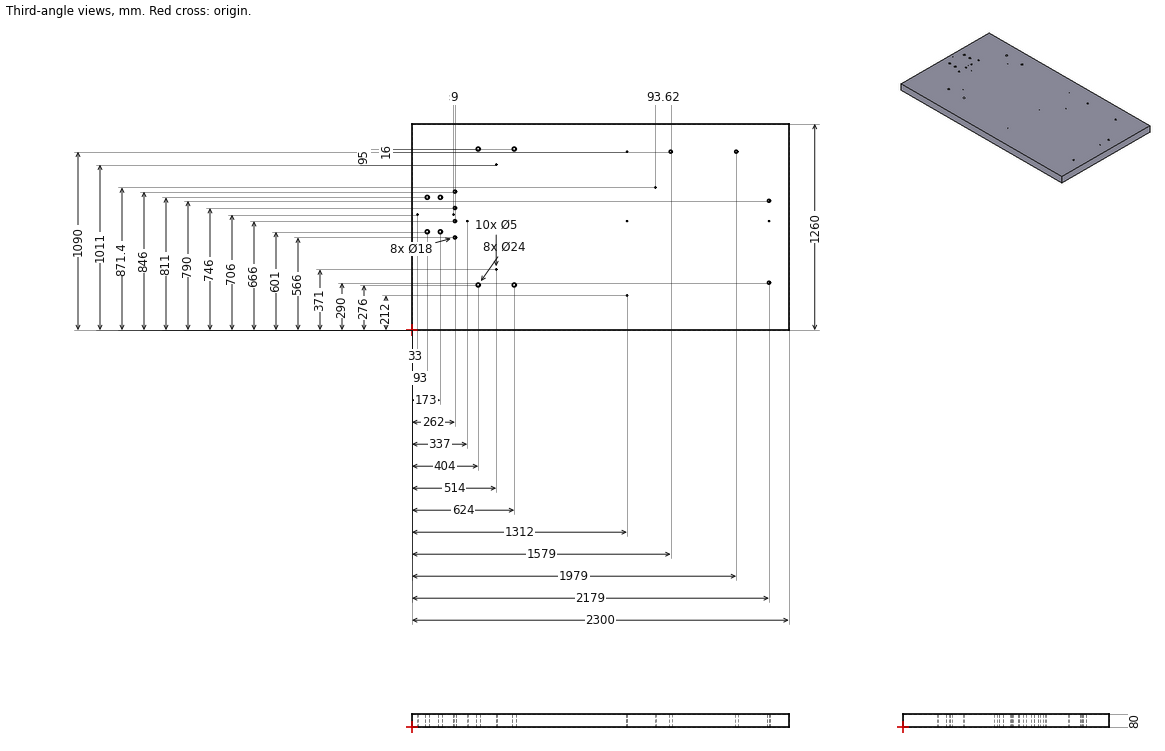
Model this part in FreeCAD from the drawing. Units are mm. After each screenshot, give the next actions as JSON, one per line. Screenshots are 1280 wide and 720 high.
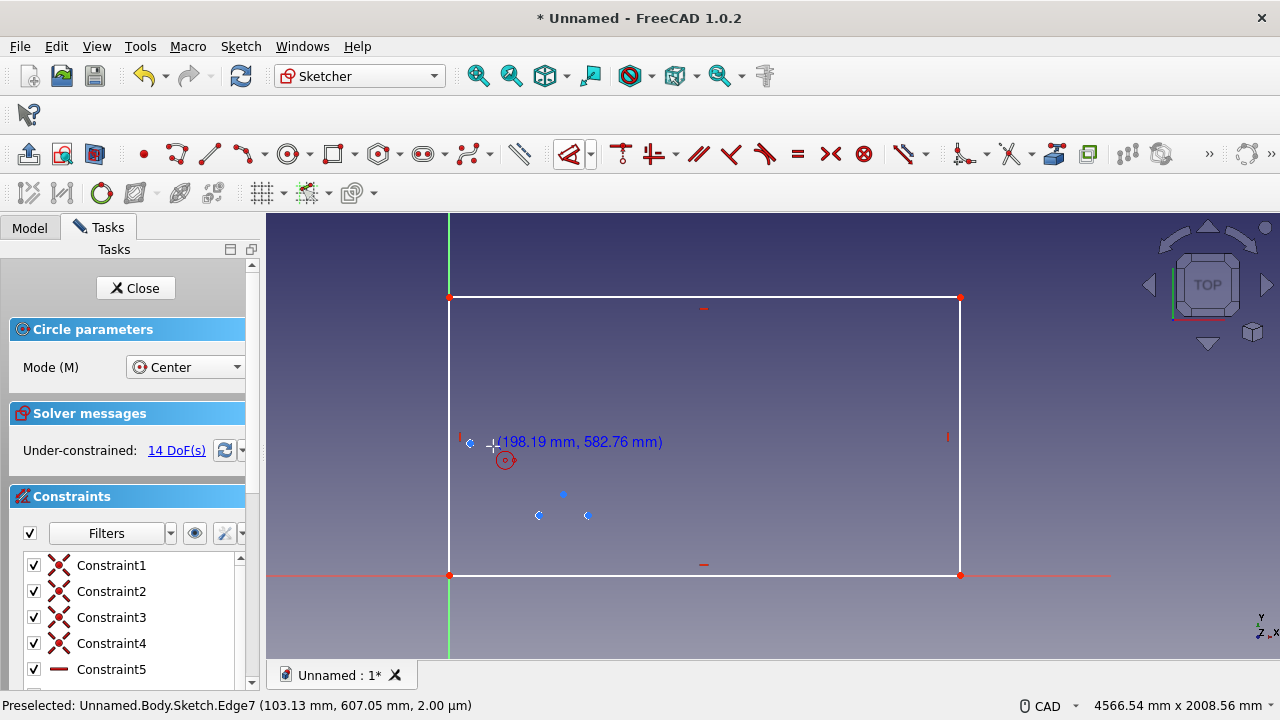
{"action": "left_click", "coordinate": [507, 450]}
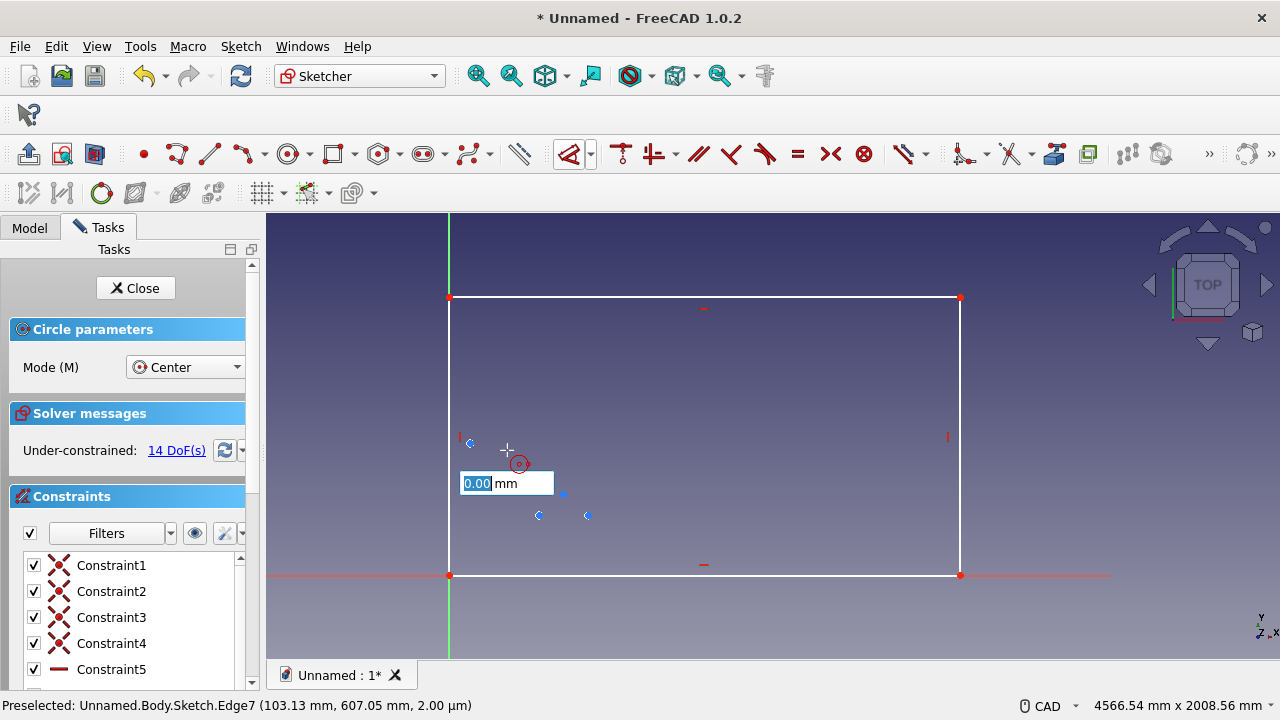
{"action": "scroll", "coordinate": [509, 449], "scroll_direction": "up", "scroll_amount": 11}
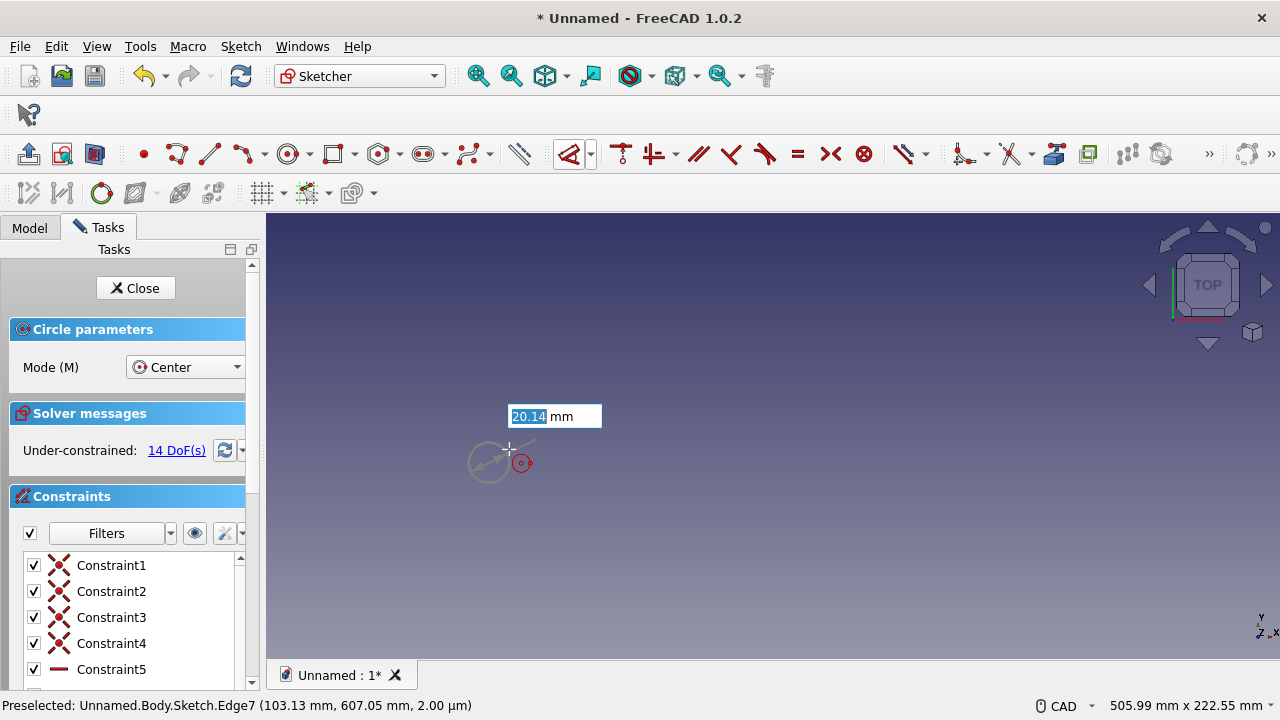
{"action": "left_click", "coordinate": [505, 444]}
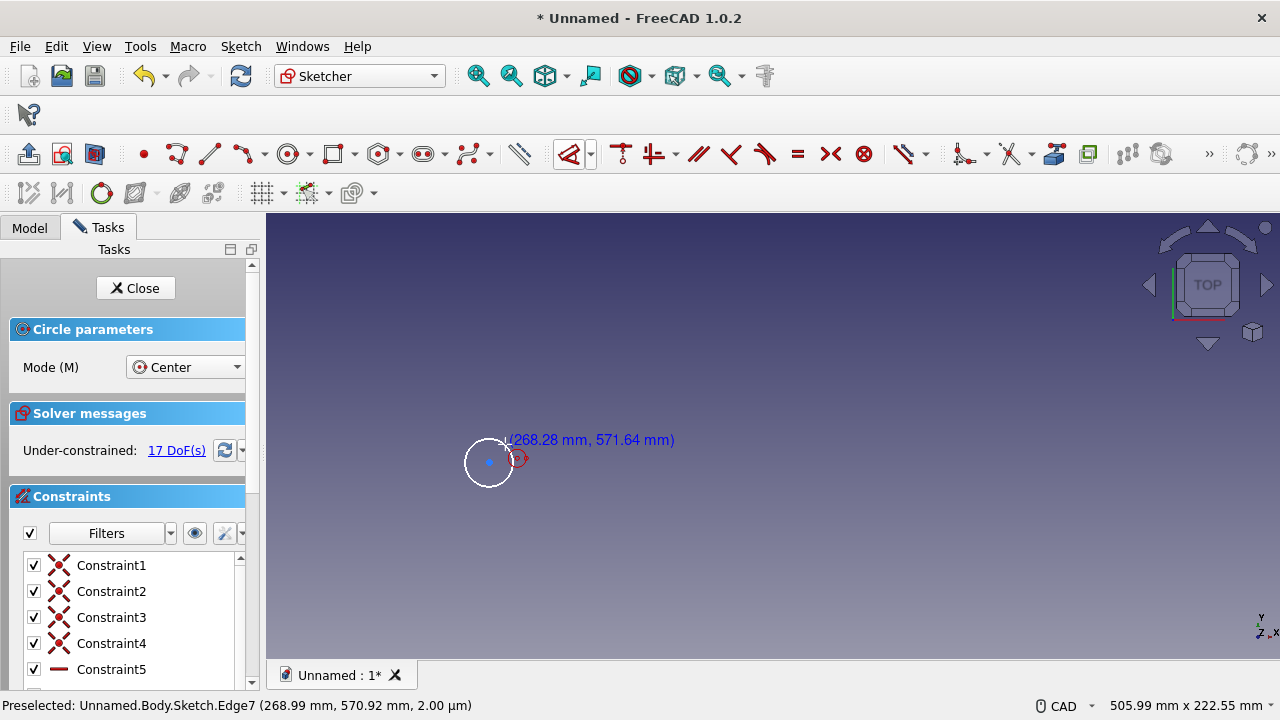
{"action": "scroll", "coordinate": [509, 449], "scroll_direction": "down", "scroll_amount": 11}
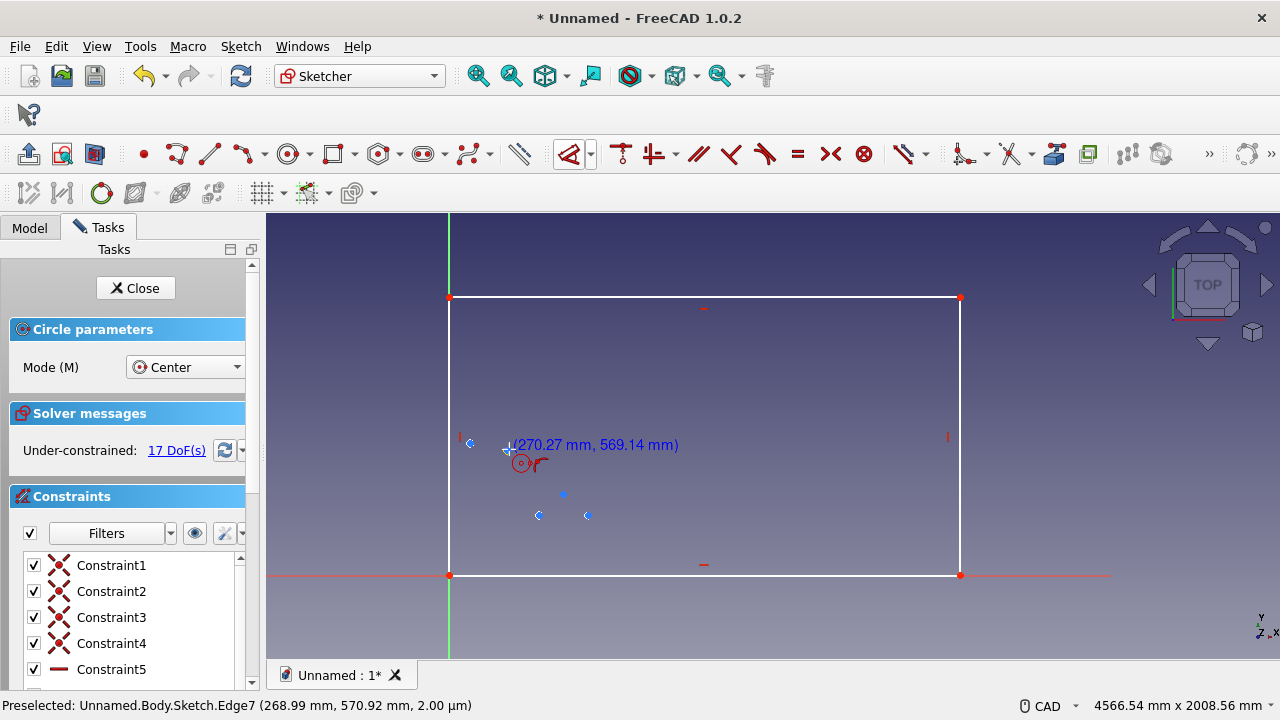
{"action": "left_click", "coordinate": [488, 443]}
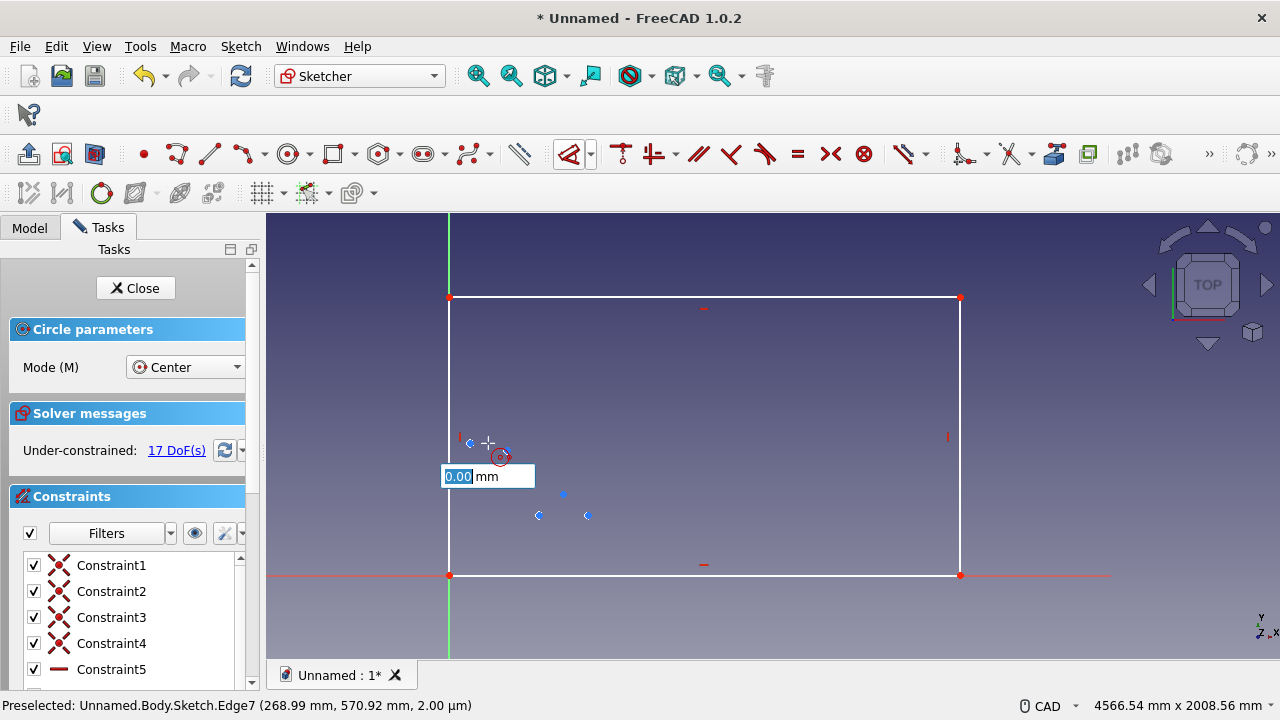
{"action": "scroll", "coordinate": [489, 441], "scroll_direction": "up", "scroll_amount": 9}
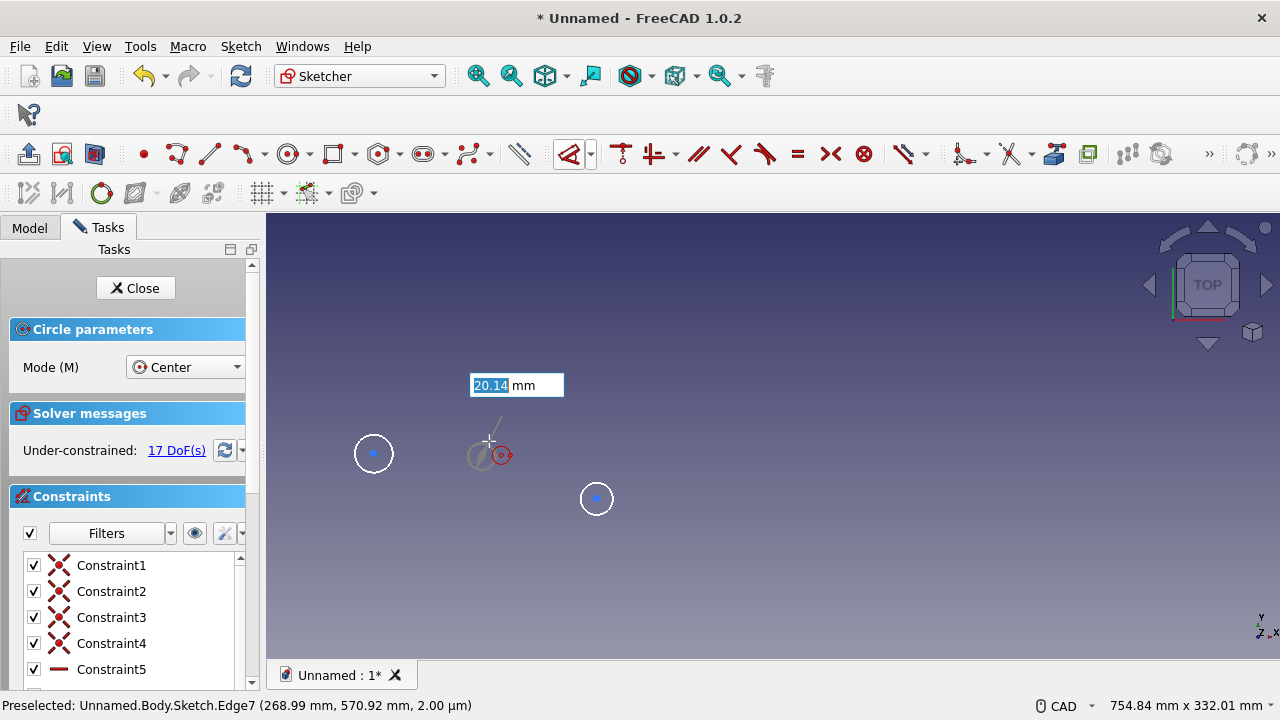
{"action": "left_click", "coordinate": [491, 436]}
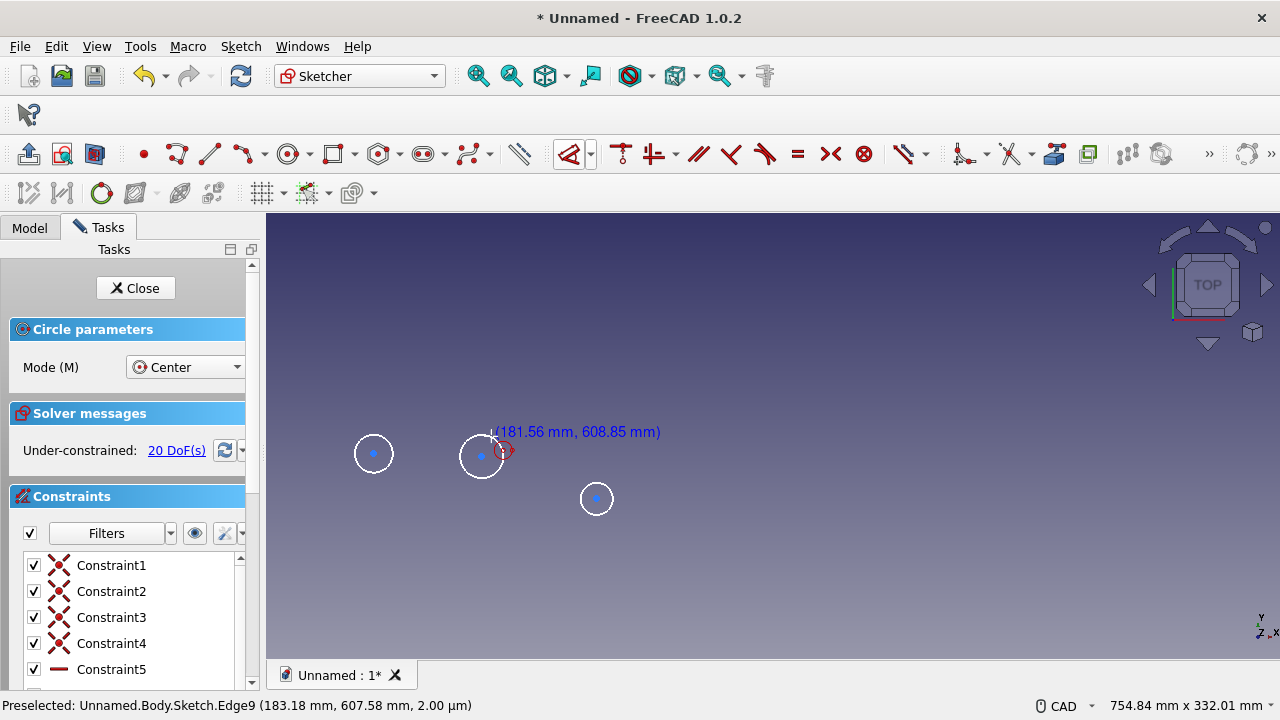
{"action": "scroll", "coordinate": [489, 441], "scroll_direction": "down", "scroll_amount": 9}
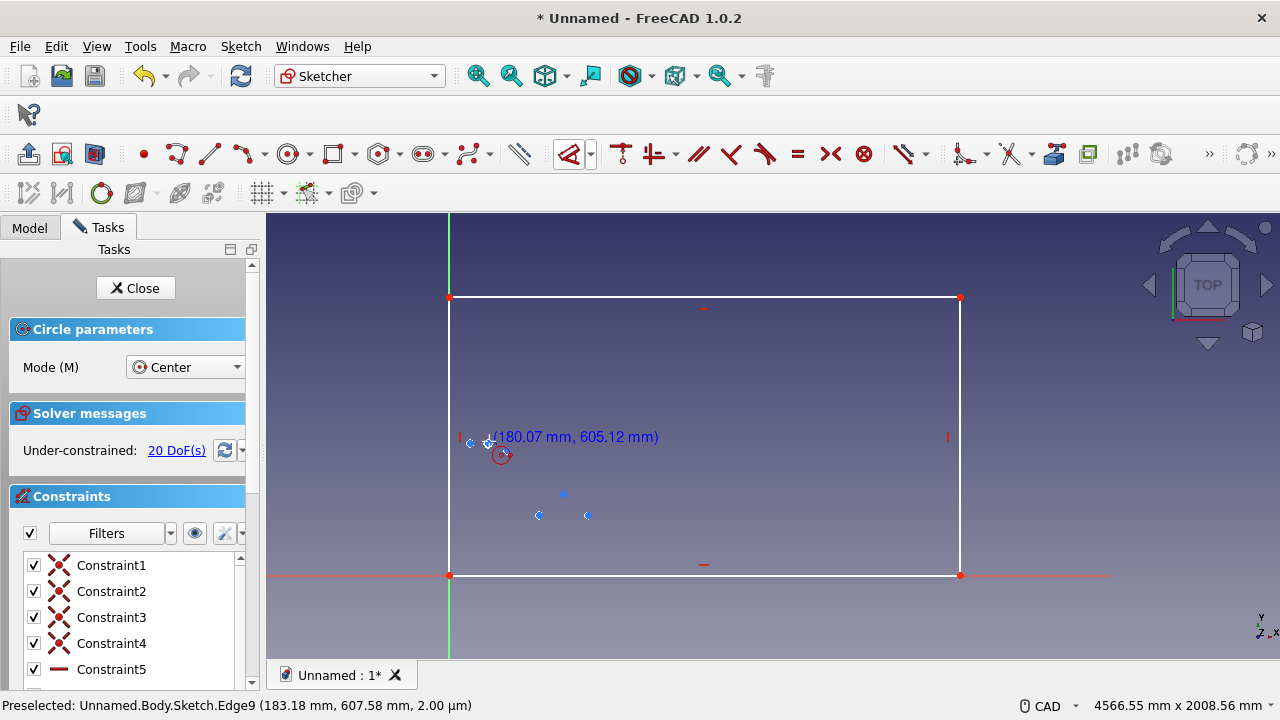
{"action": "scroll", "coordinate": [741, 529], "scroll_direction": "up", "scroll_amount": 19}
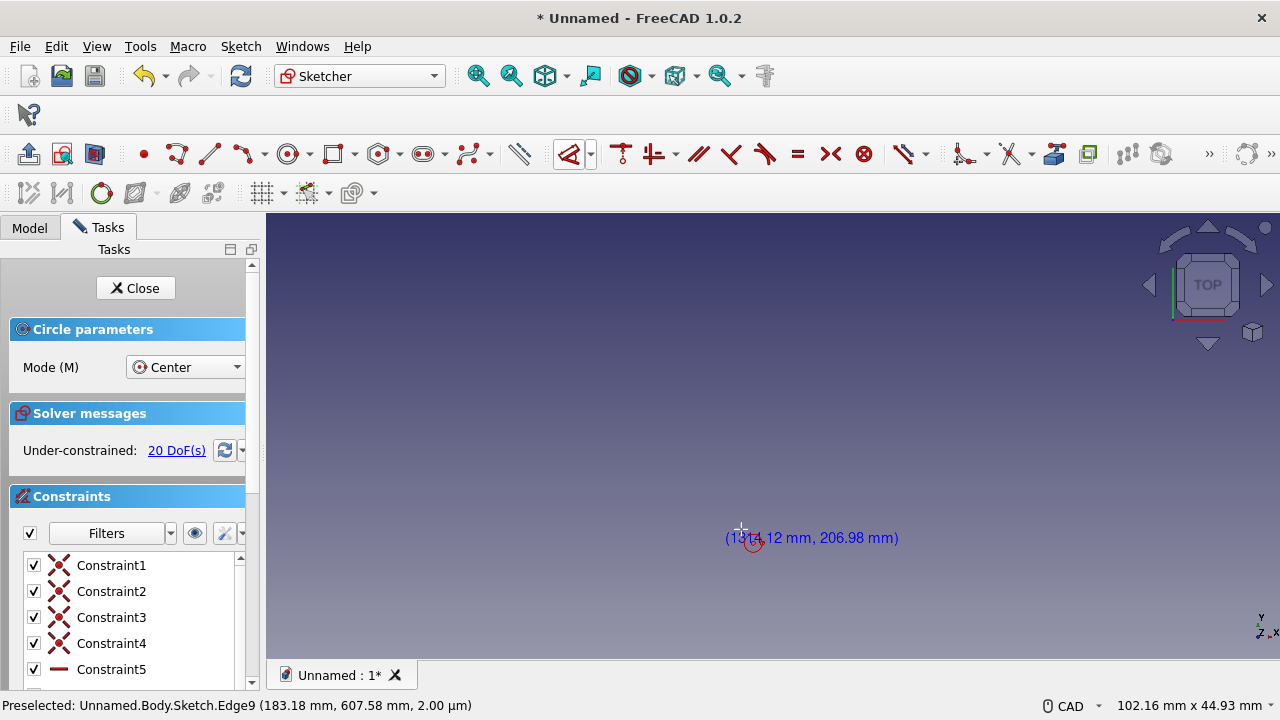
{"action": "scroll", "coordinate": [704, 436], "scroll_direction": "down", "scroll_amount": 15}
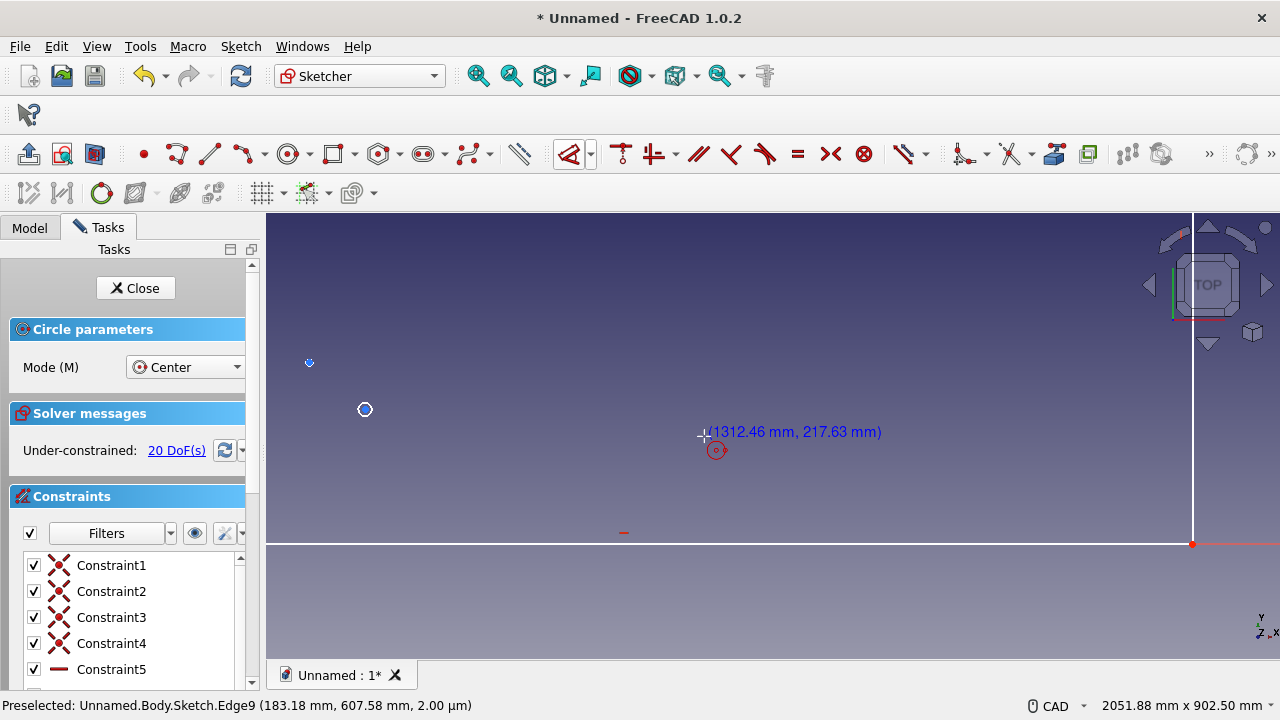
{"action": "scroll", "coordinate": [770, 602], "scroll_direction": "down", "scroll_amount": 4}